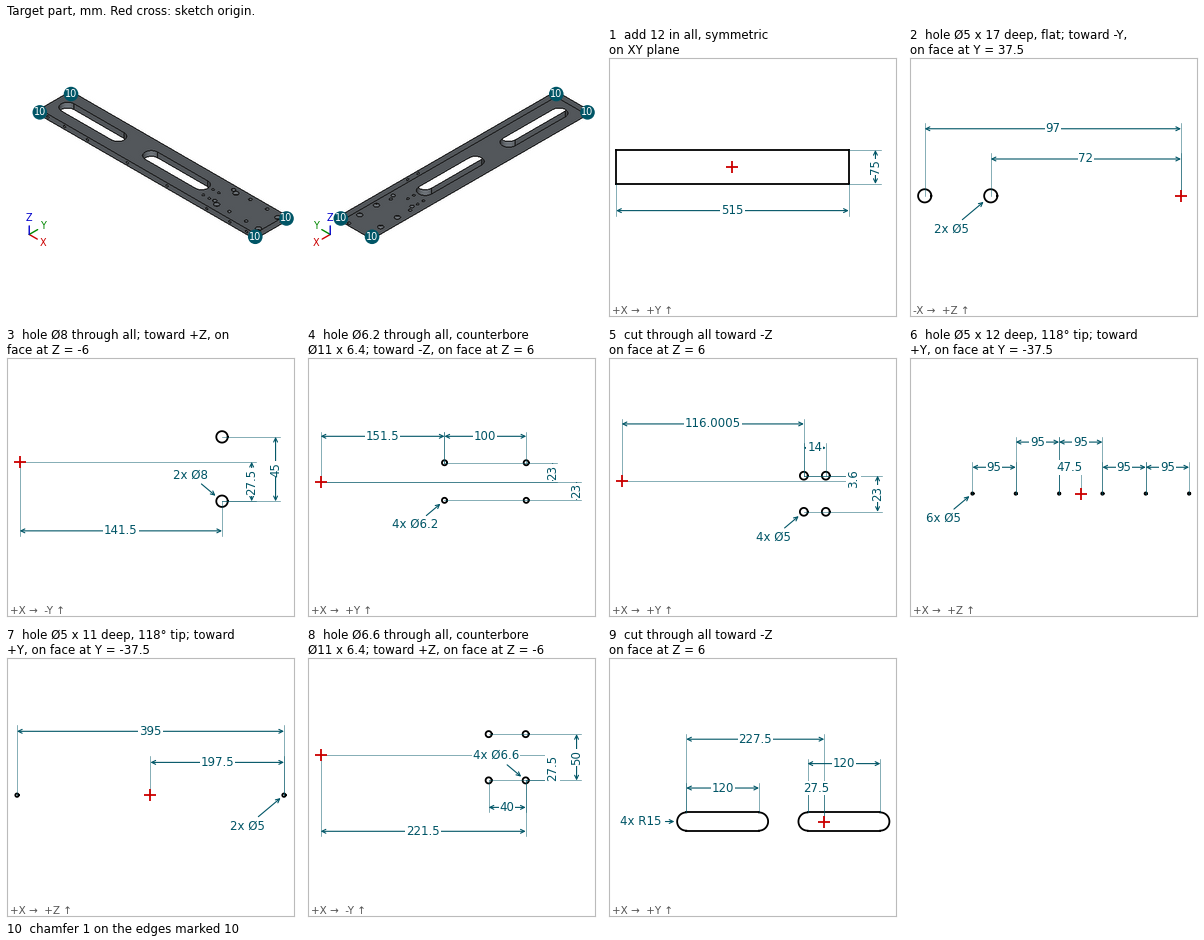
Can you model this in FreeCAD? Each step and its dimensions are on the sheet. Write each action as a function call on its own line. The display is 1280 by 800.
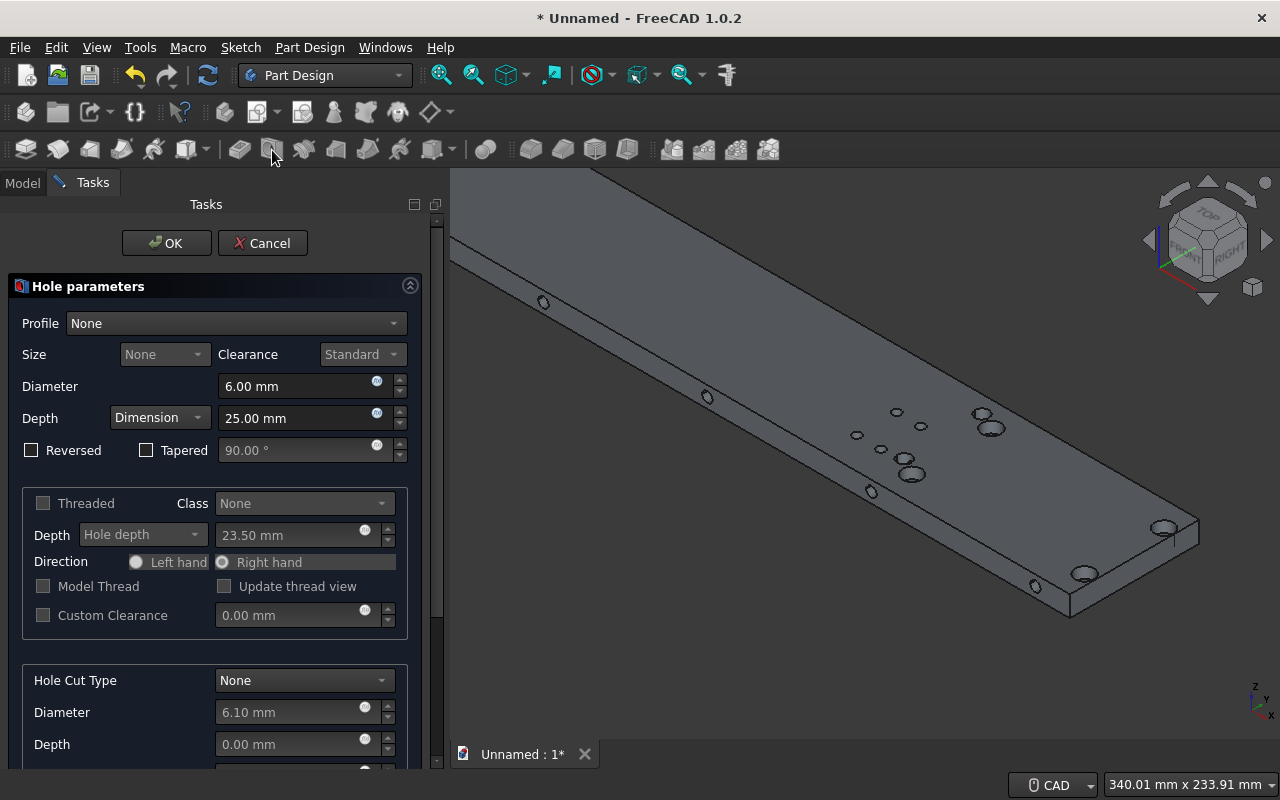
triple_click(305, 386)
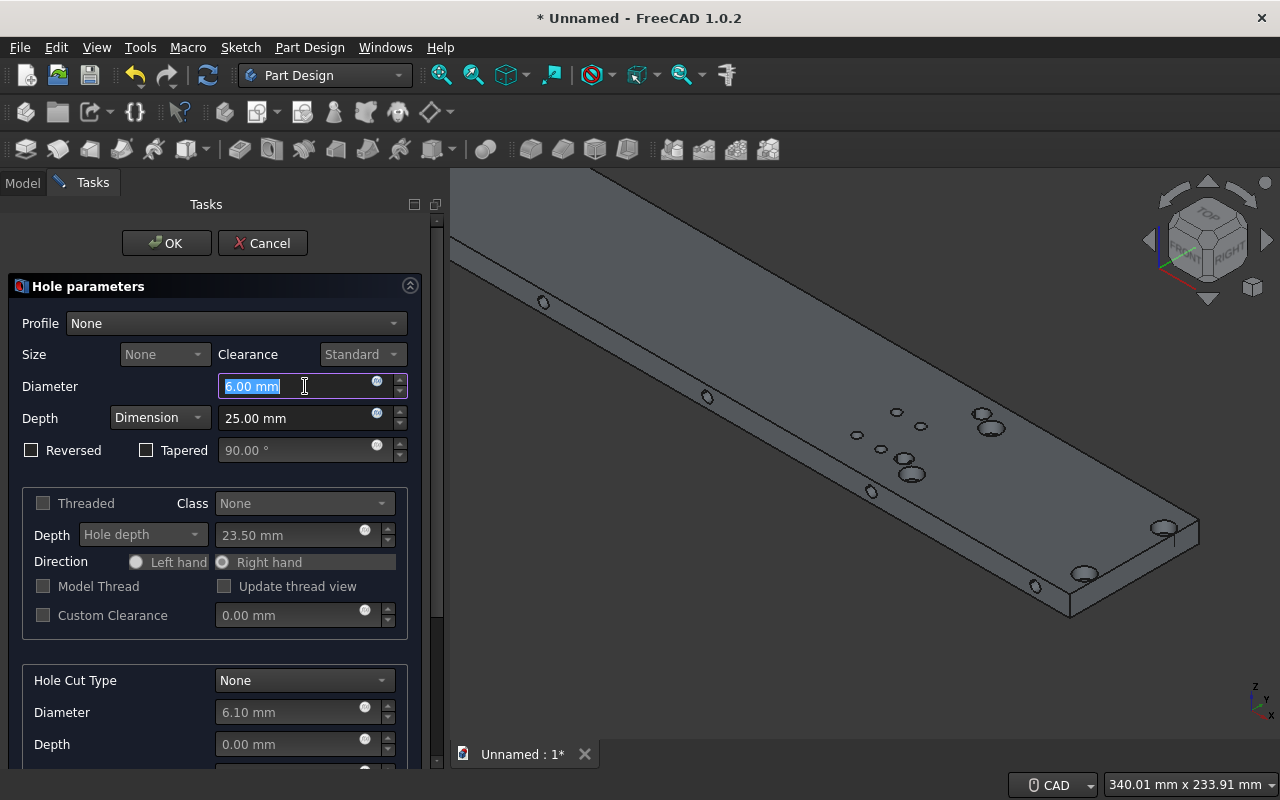
text(5)
key(Tab)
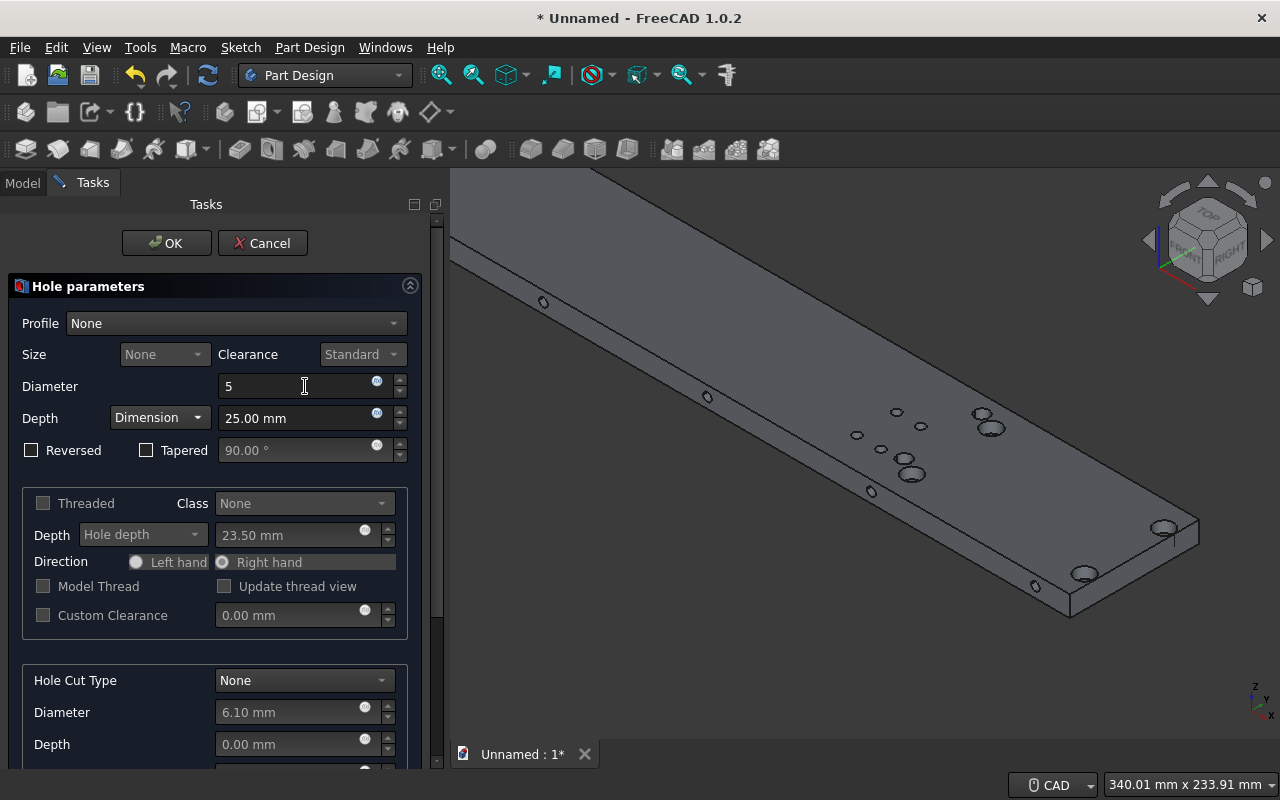
triple_click(305, 418)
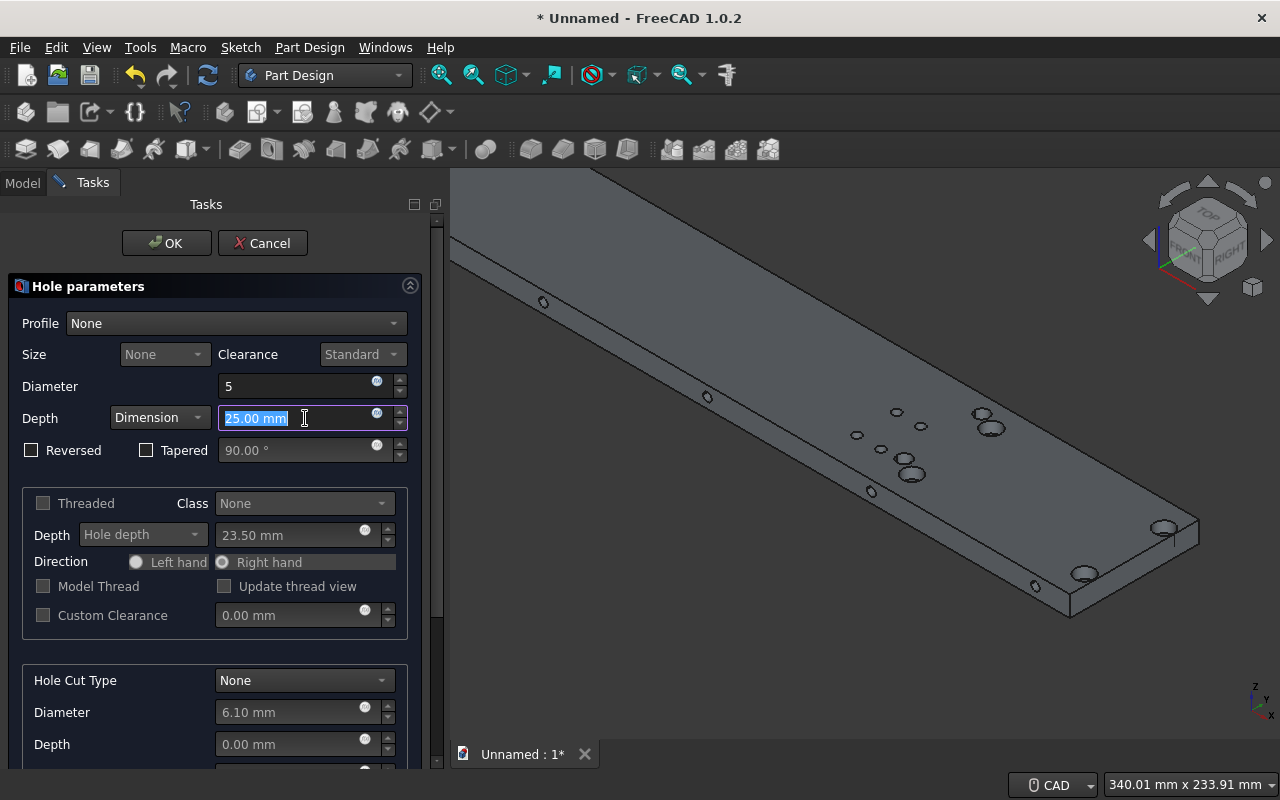
text(12)
key(Tab)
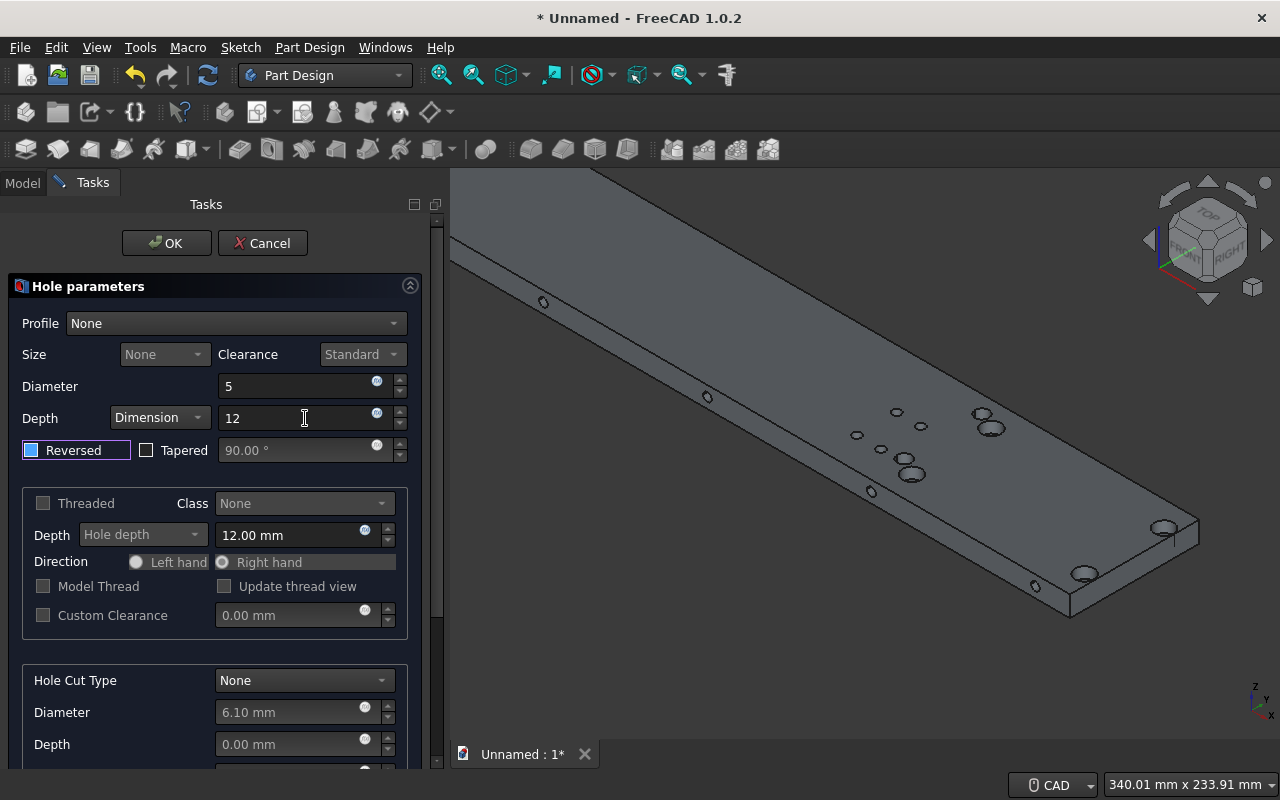
click(167, 243)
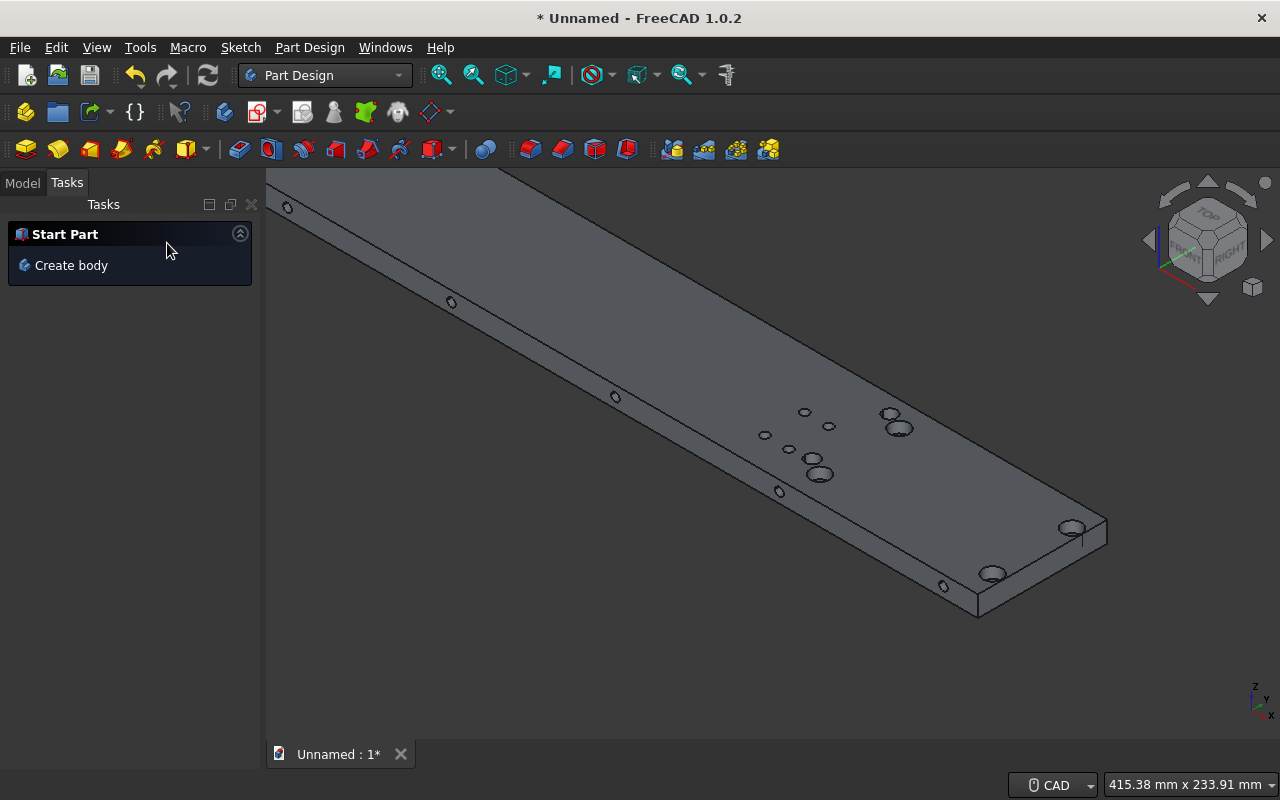
key(v)
key(f)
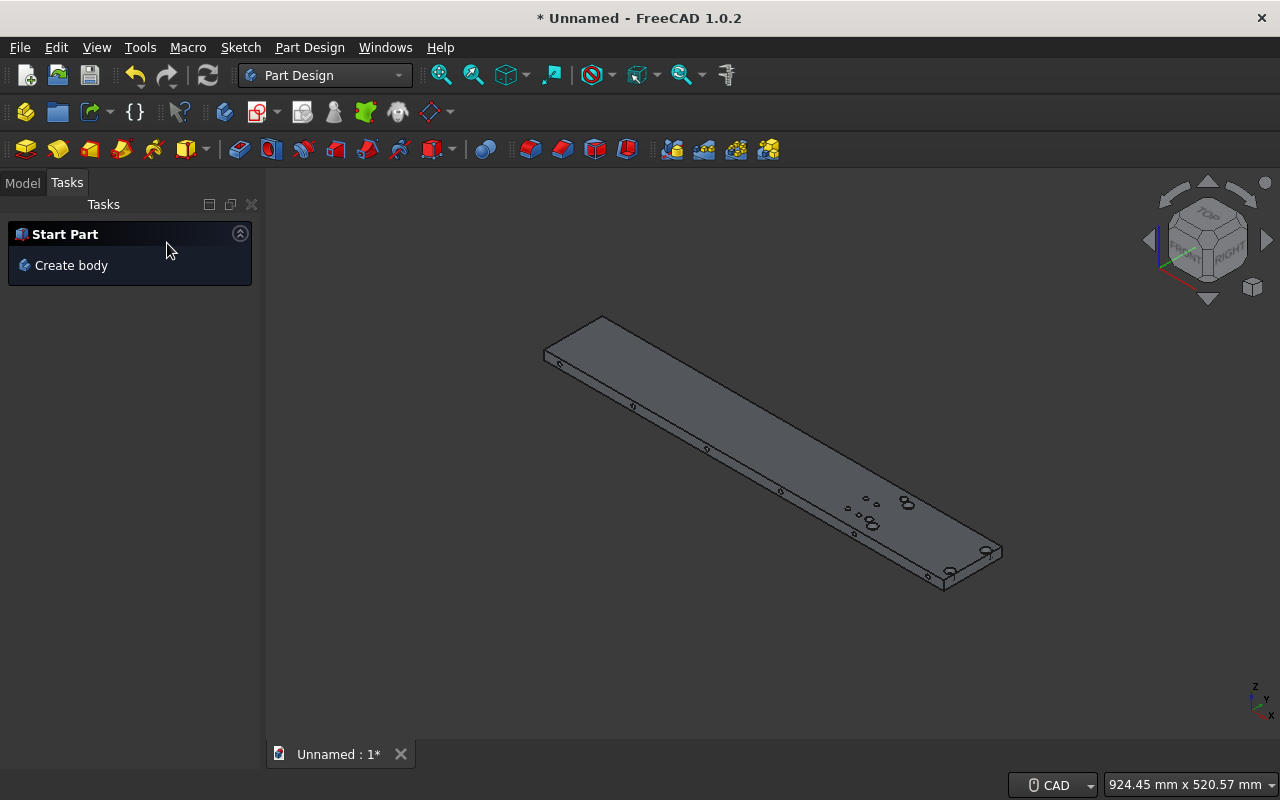
scroll(915, 568, up, 4)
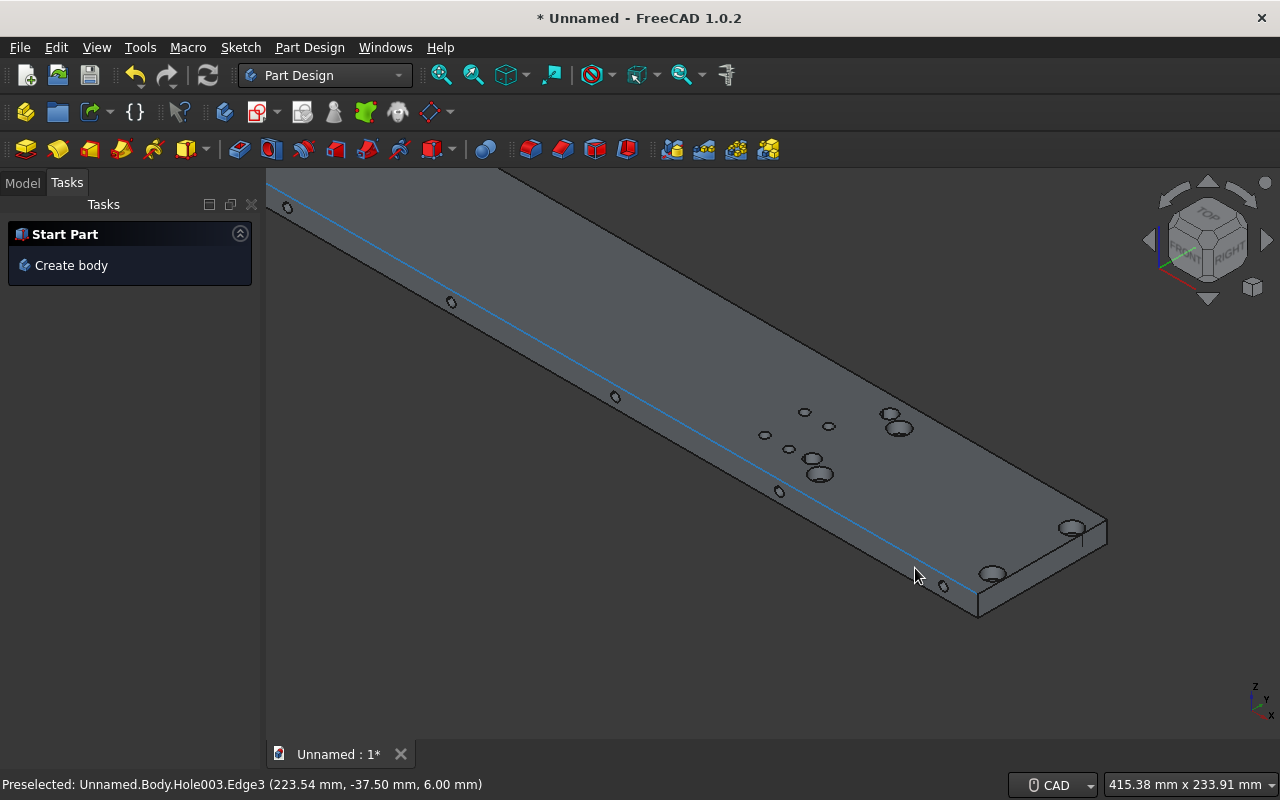
click(914, 569)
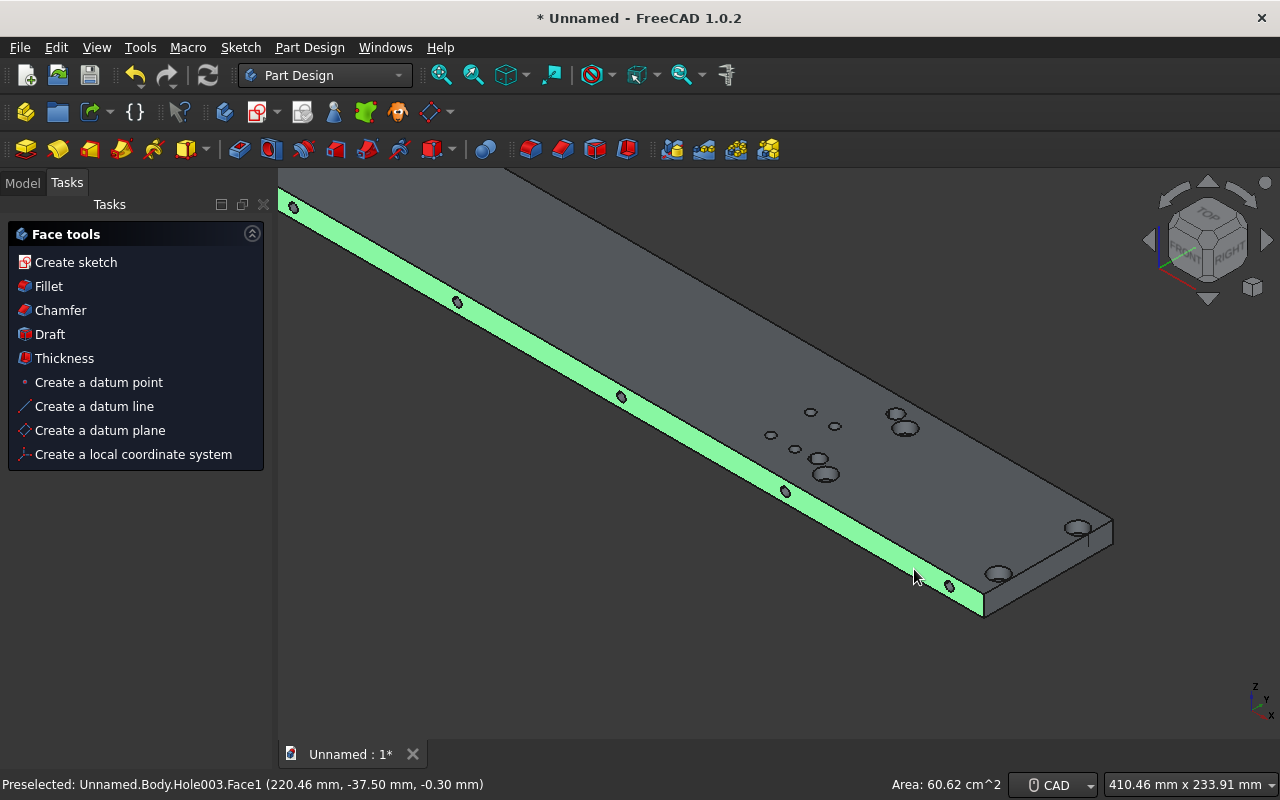
click(258, 112)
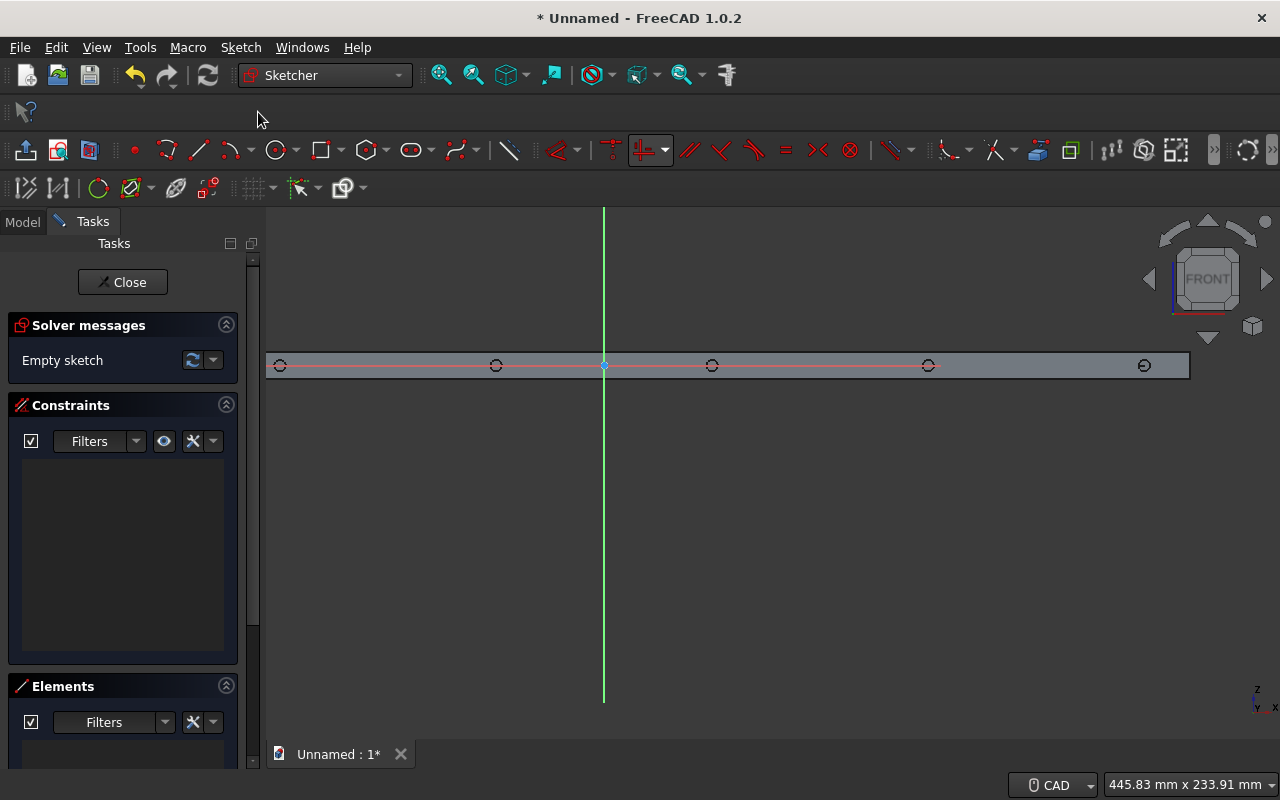
scroll(909, 691, down, 2)